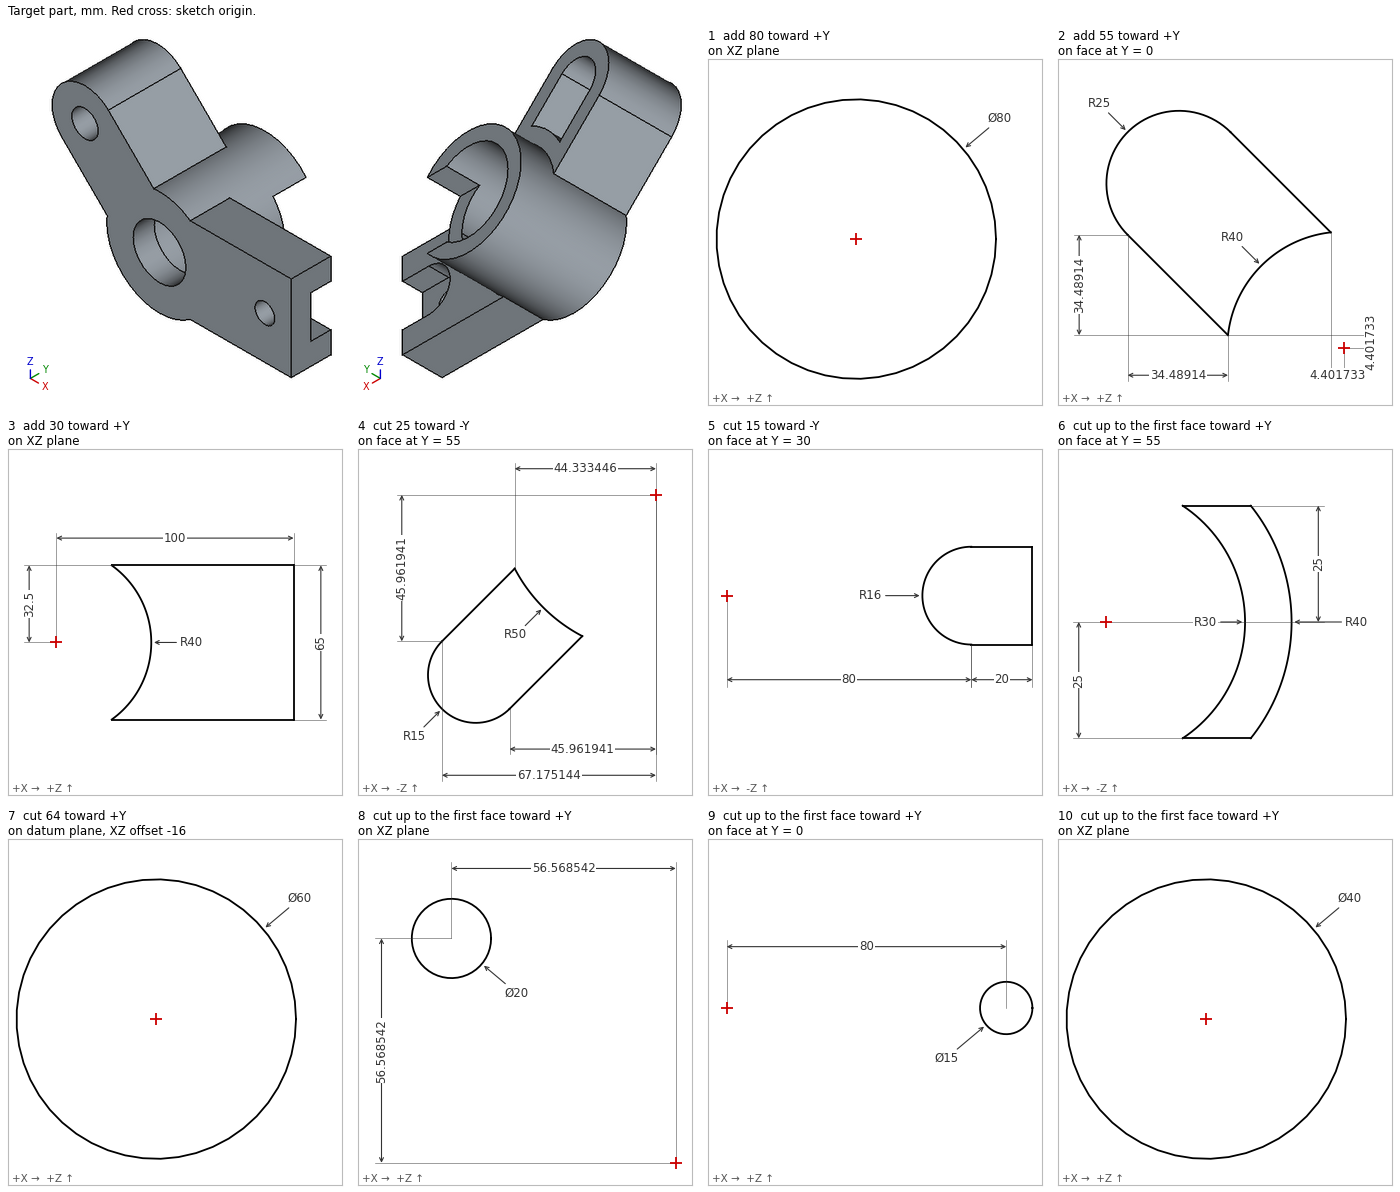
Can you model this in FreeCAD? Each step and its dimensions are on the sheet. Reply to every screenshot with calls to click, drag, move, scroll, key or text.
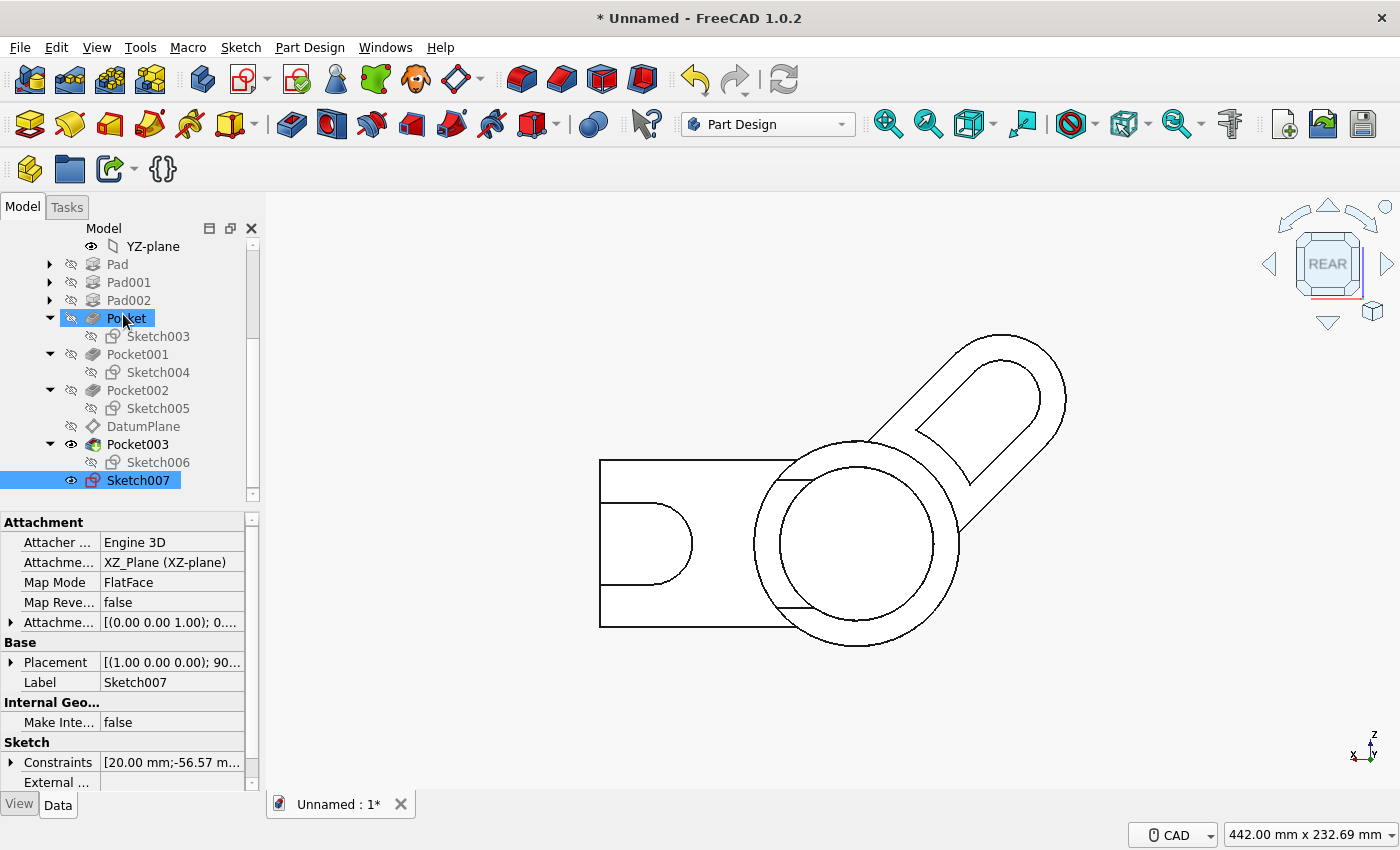
click(292, 124)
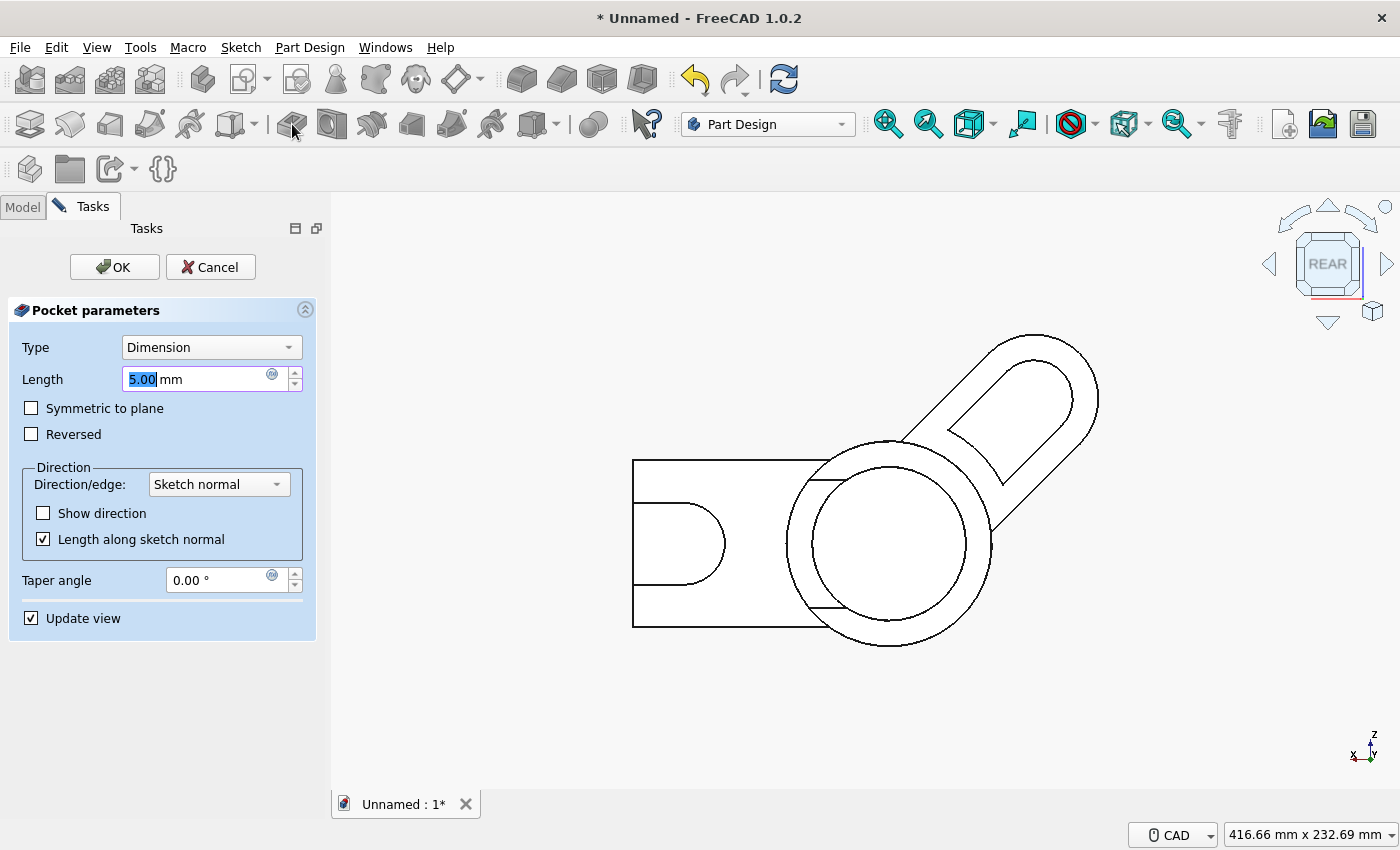
click(212, 348)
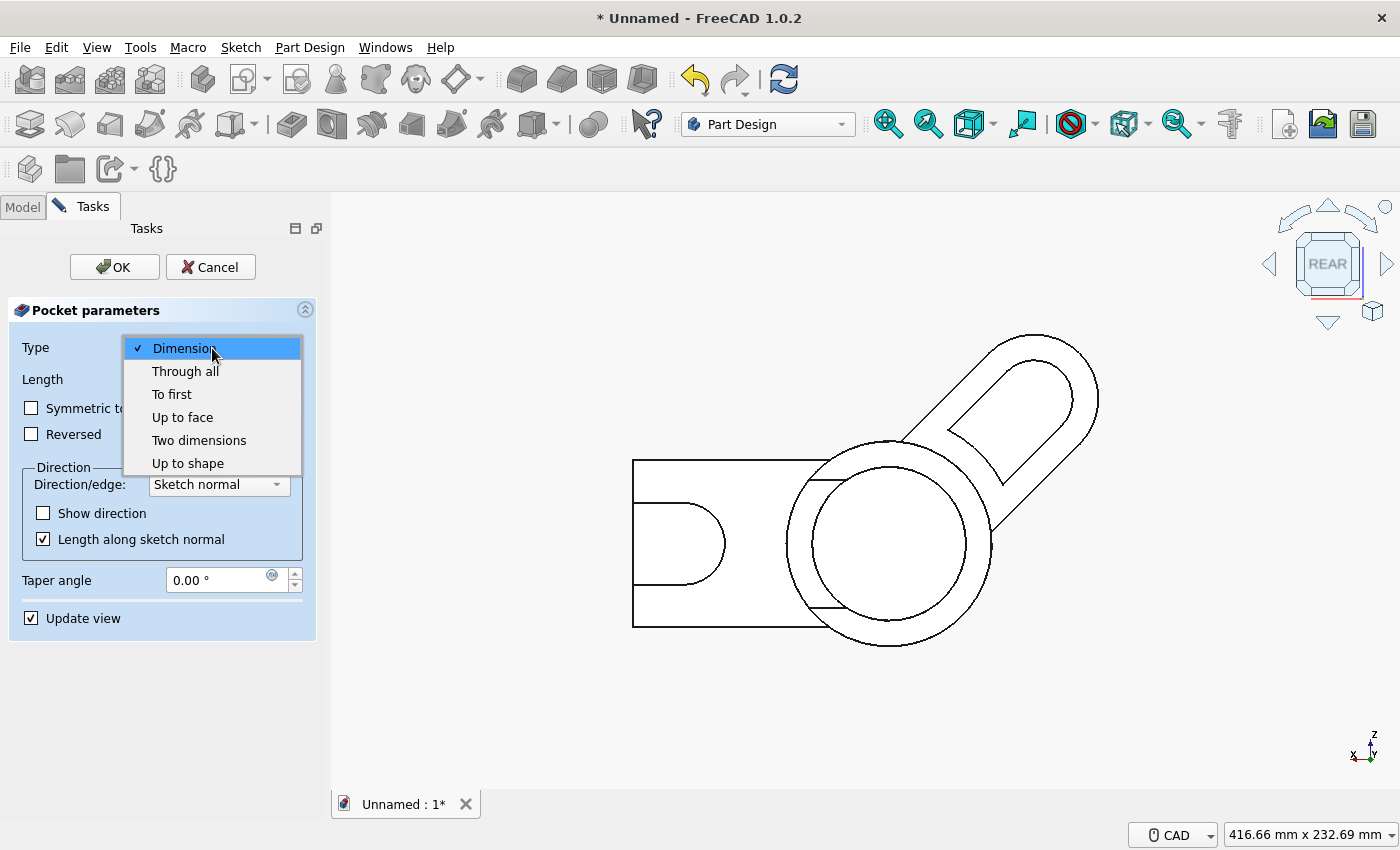
click(212, 394)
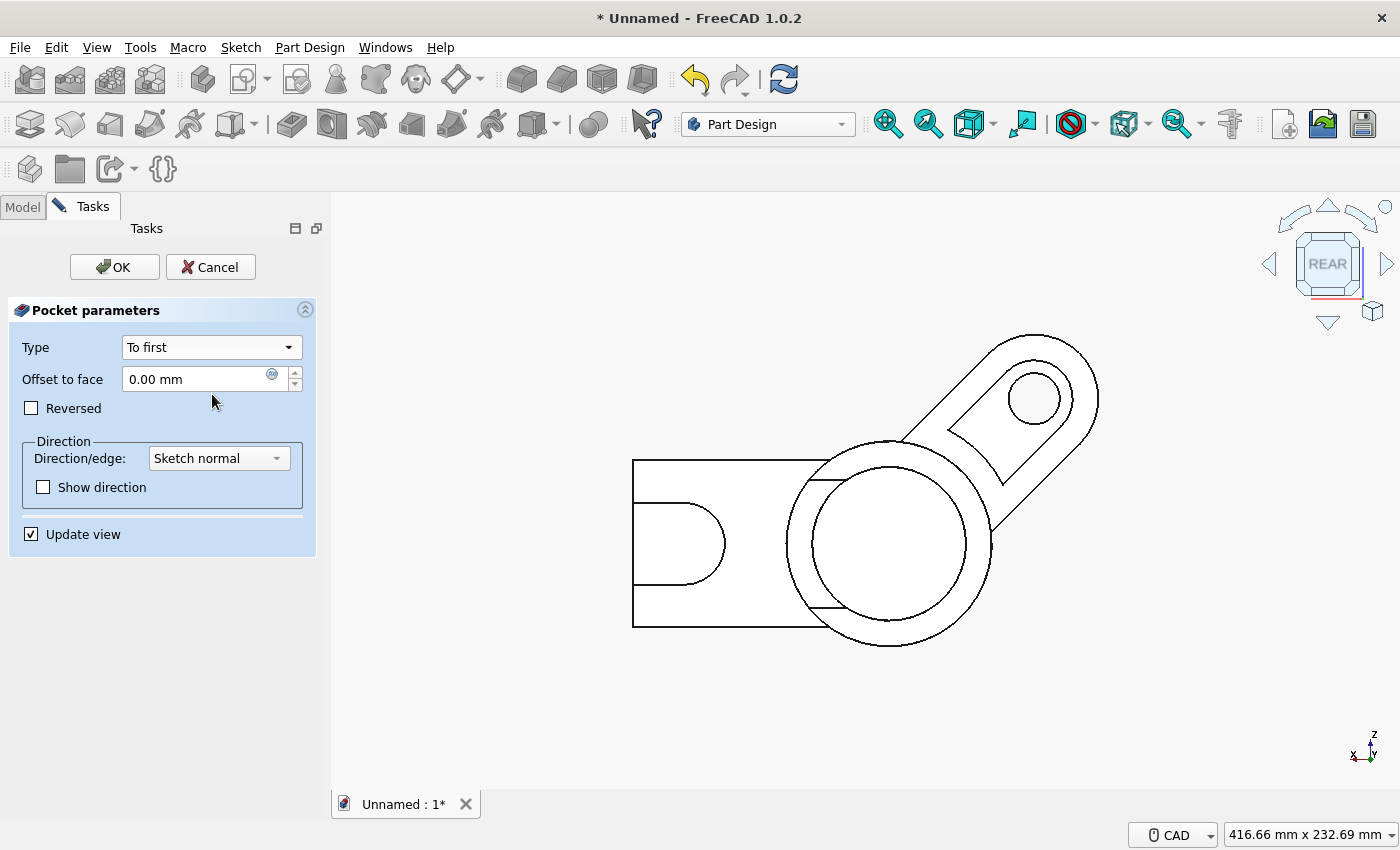
click(115, 267)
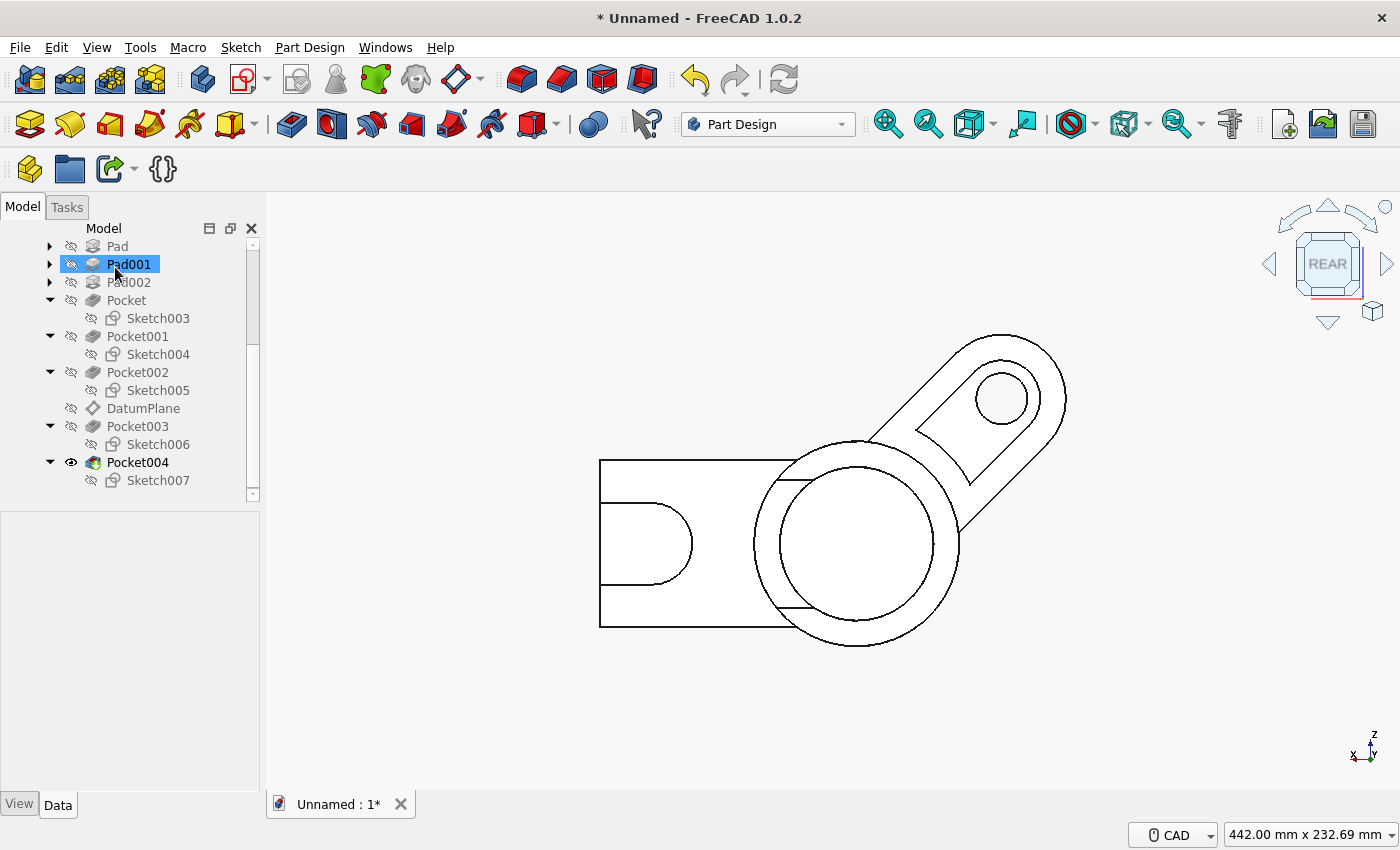
key(0)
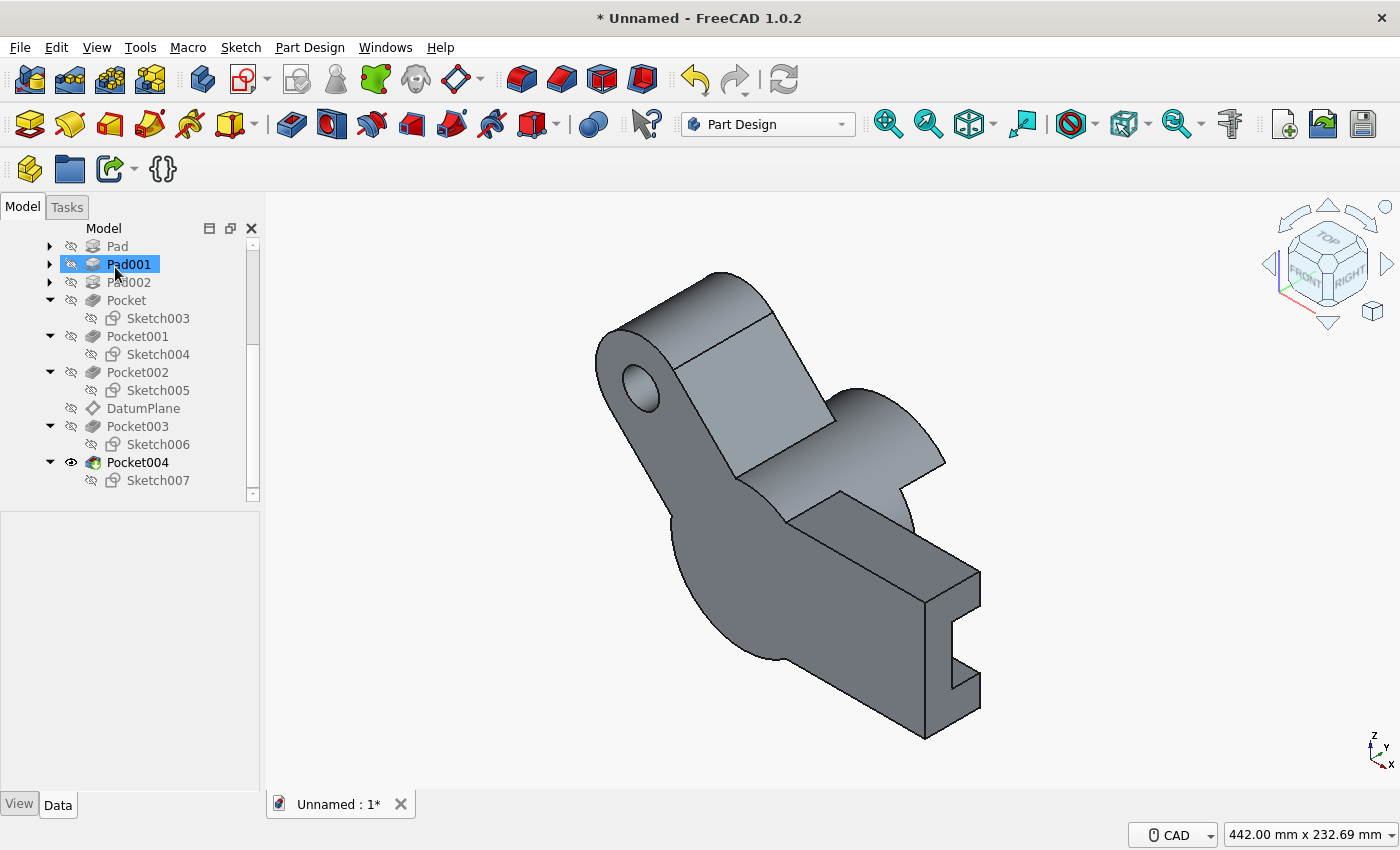
click(760, 568)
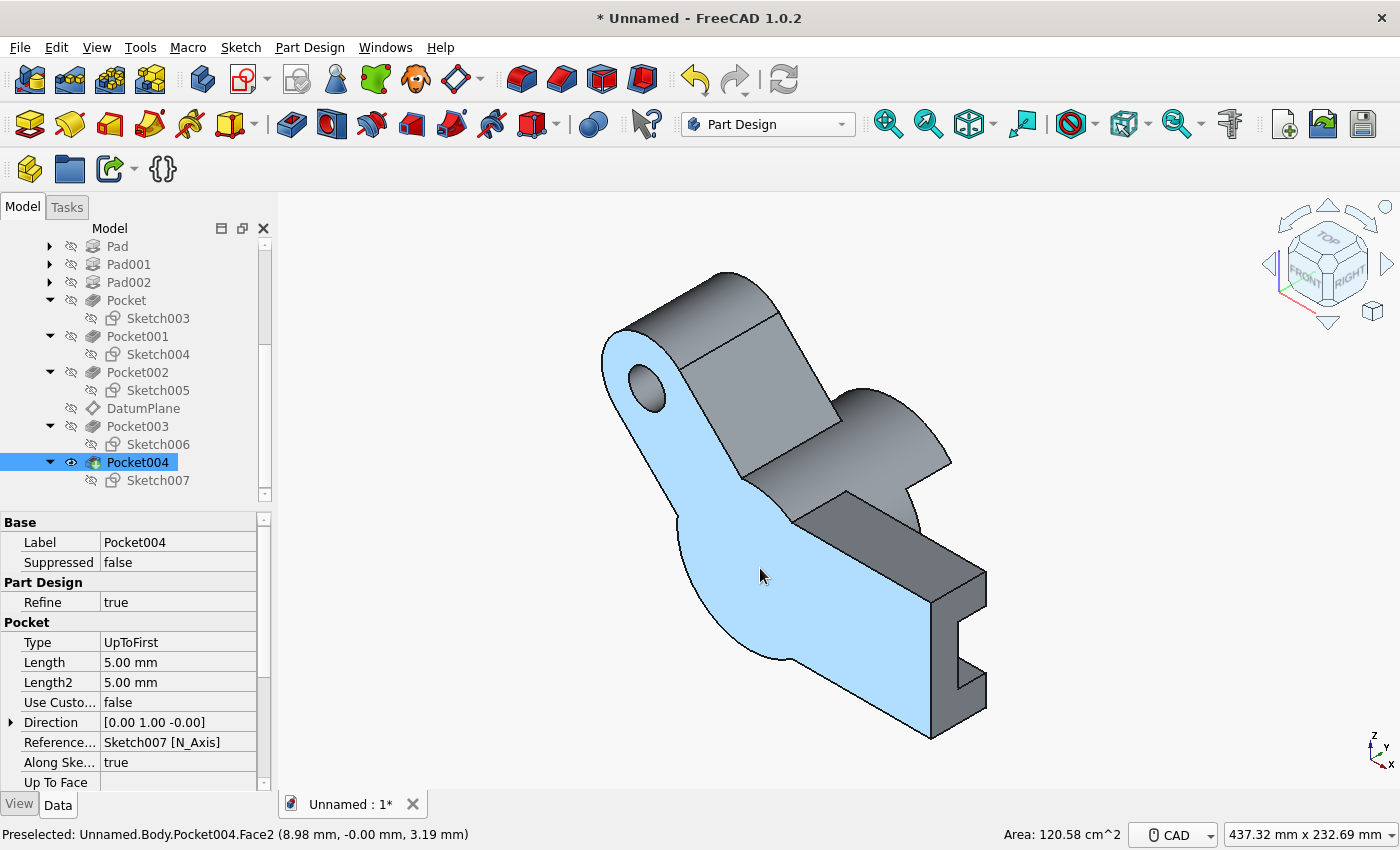
click(244, 80)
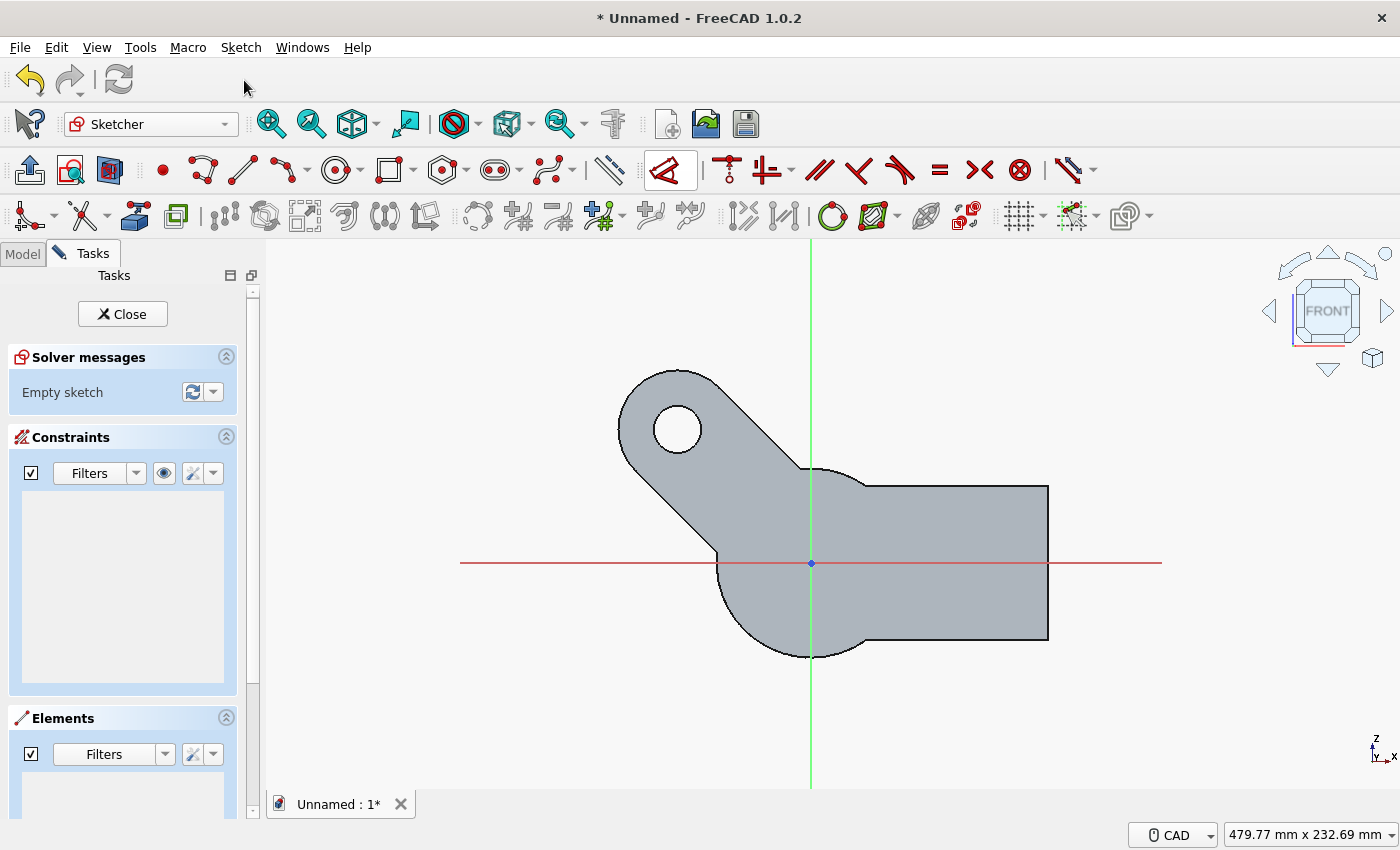
scroll(1030, 569, up, 11)